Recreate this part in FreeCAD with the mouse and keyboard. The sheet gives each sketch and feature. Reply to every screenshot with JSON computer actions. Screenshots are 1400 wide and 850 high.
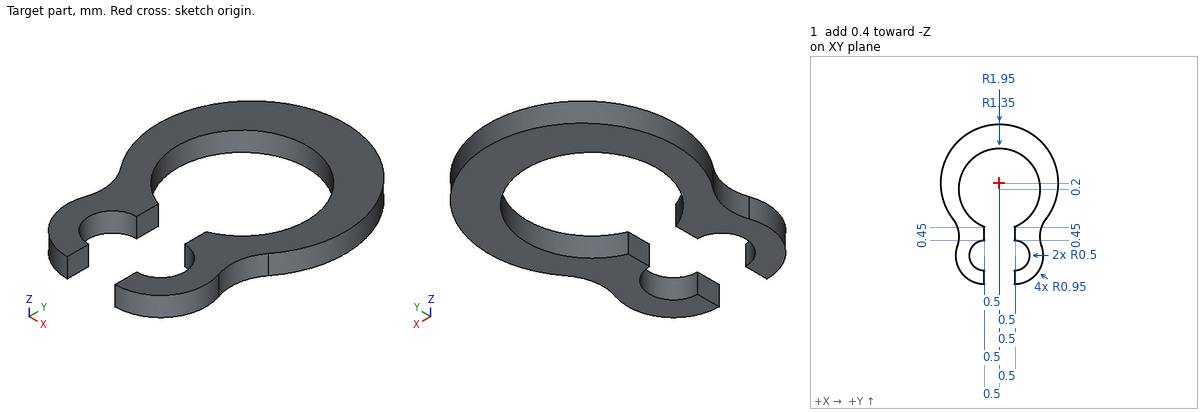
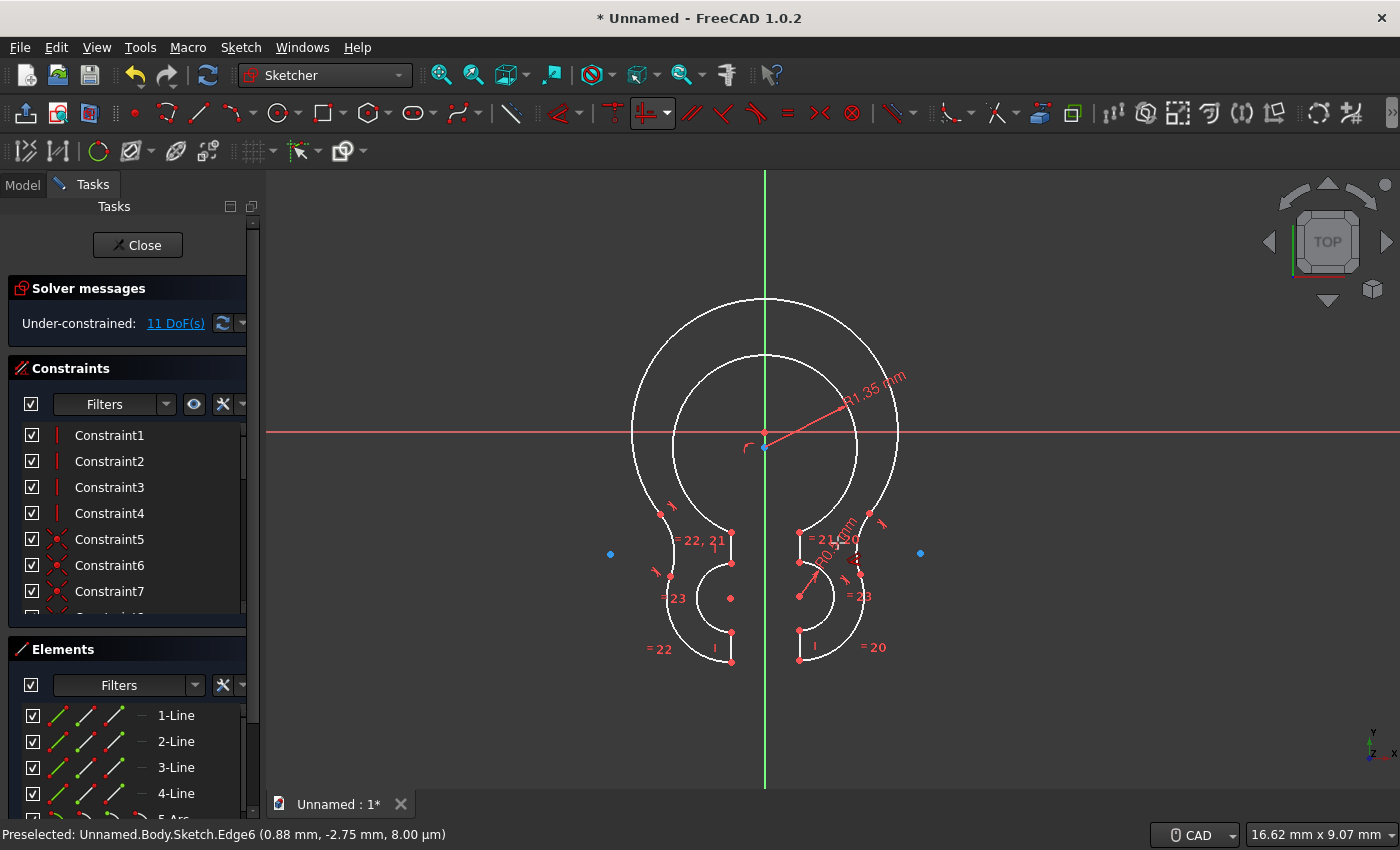
{"action": "left_click", "coordinate": [835, 650]}
{"action": "left_click", "coordinate": [853, 677]}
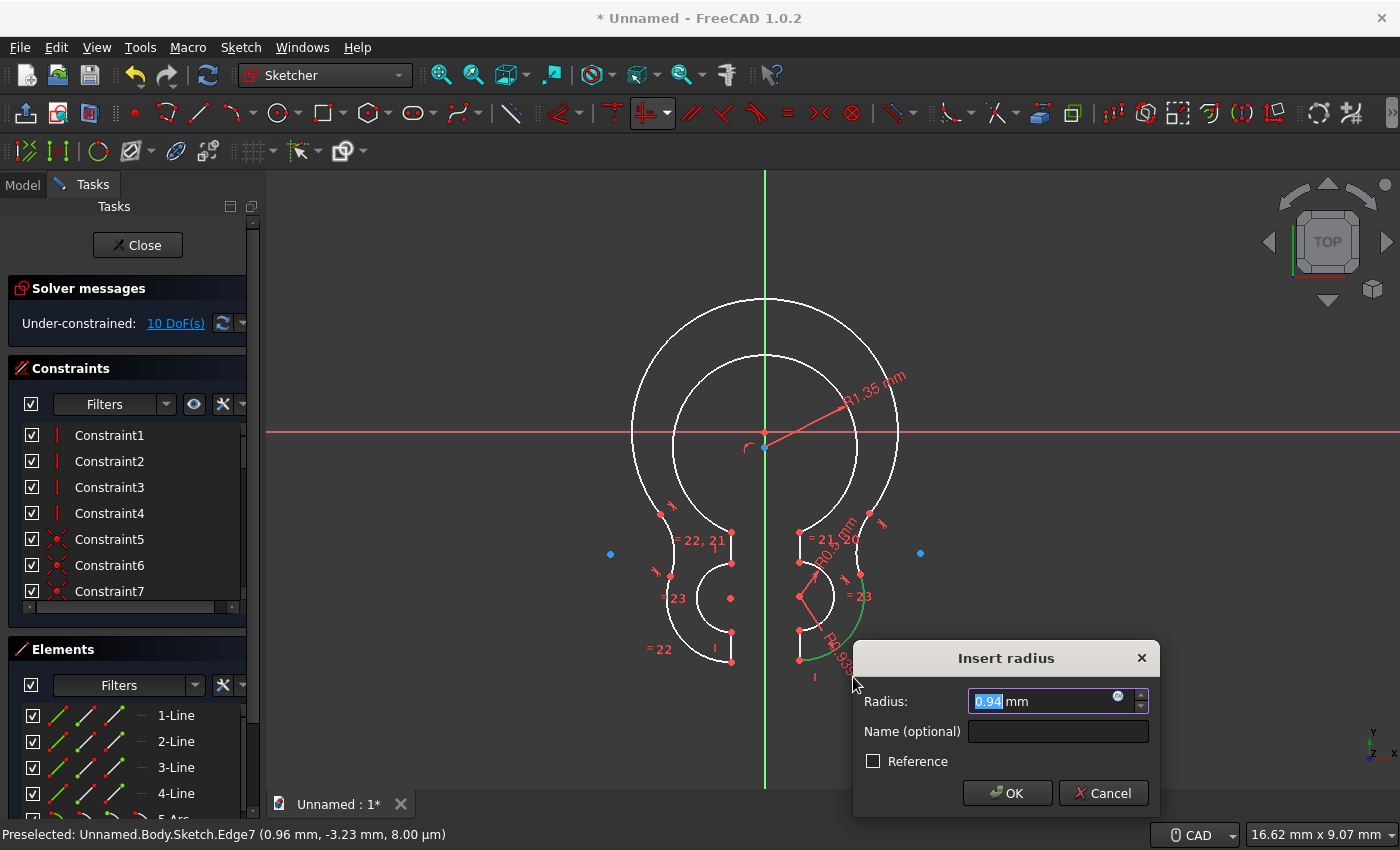
{"action": "type", "text": "0.95"}
{"action": "key", "text": "Return"}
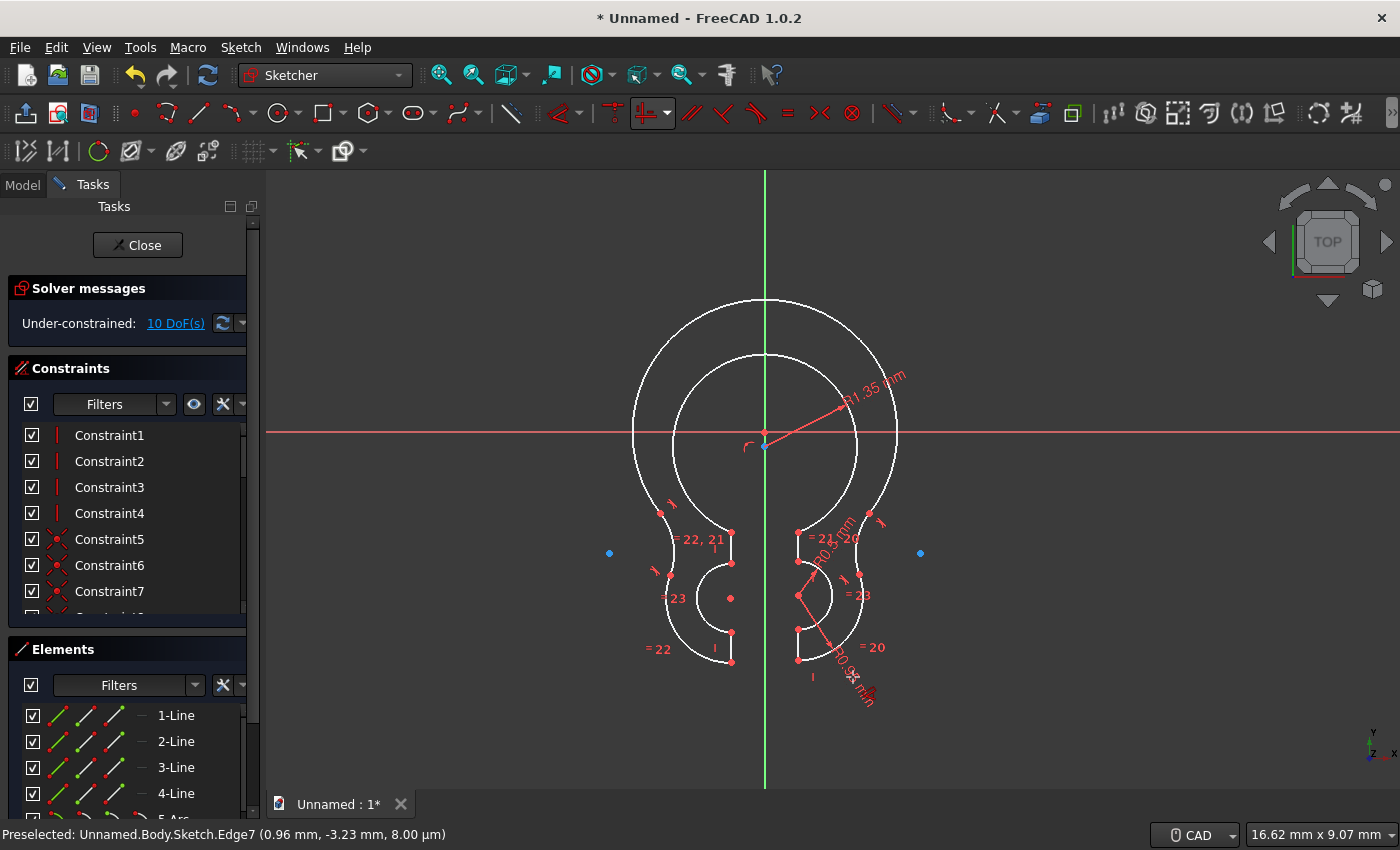
{"action": "left_click", "coordinate": [868, 349]}
{"action": "left_click", "coordinate": [893, 329]}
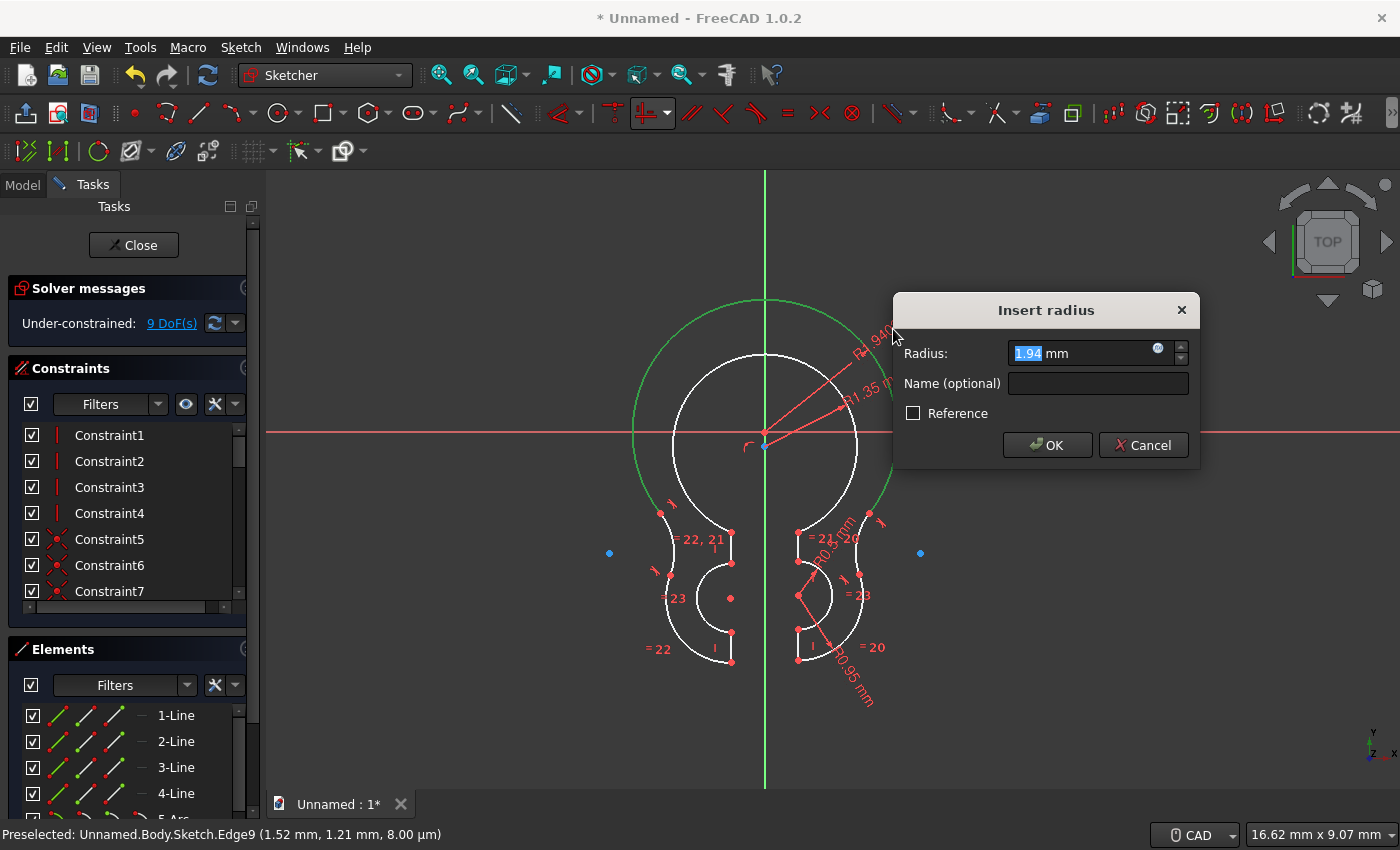
{"action": "type", "text": "1.95"}
{"action": "key", "text": "Return"}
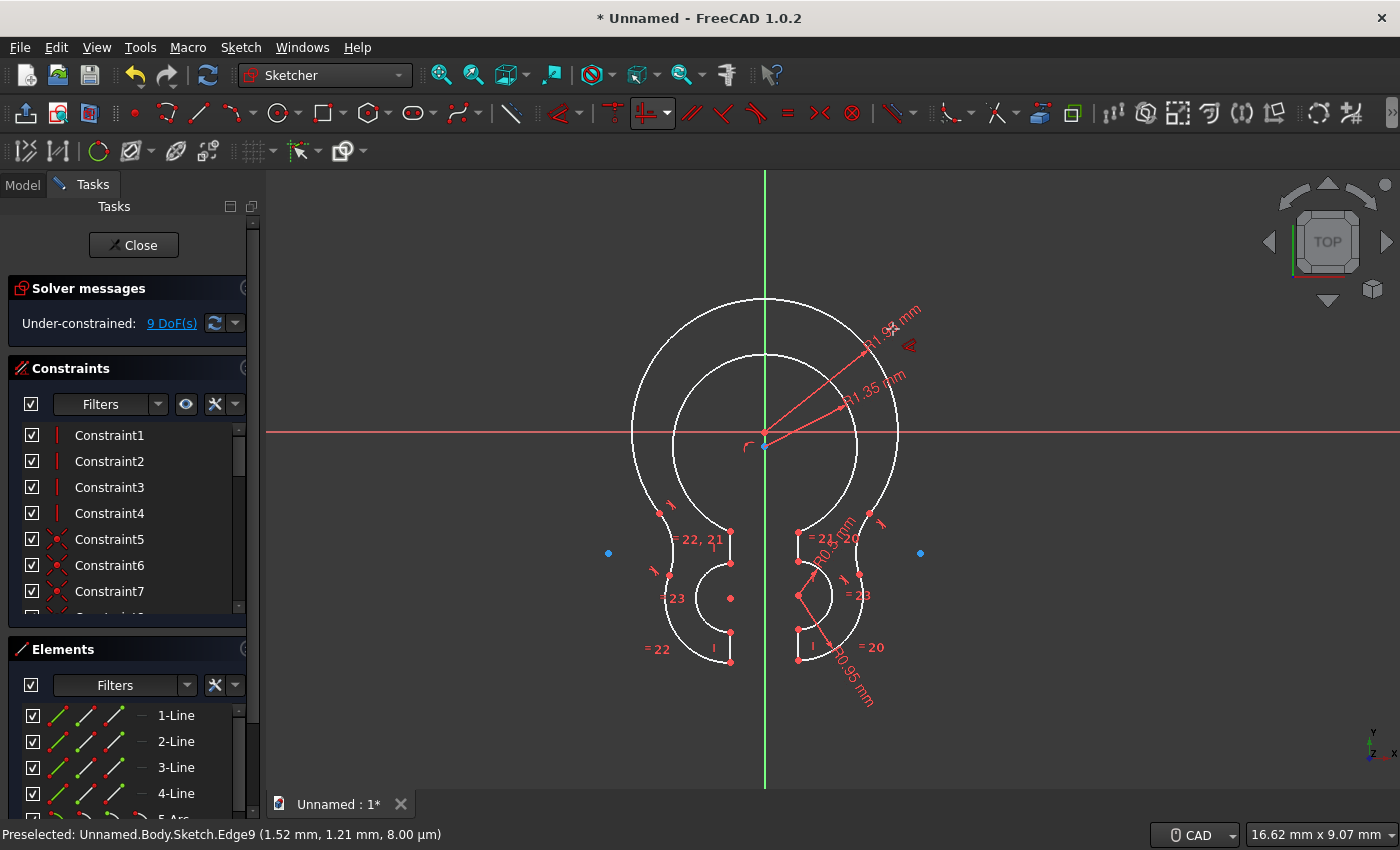
{"action": "scroll", "coordinate": [730, 554], "scroll_direction": "up", "scroll_amount": 2}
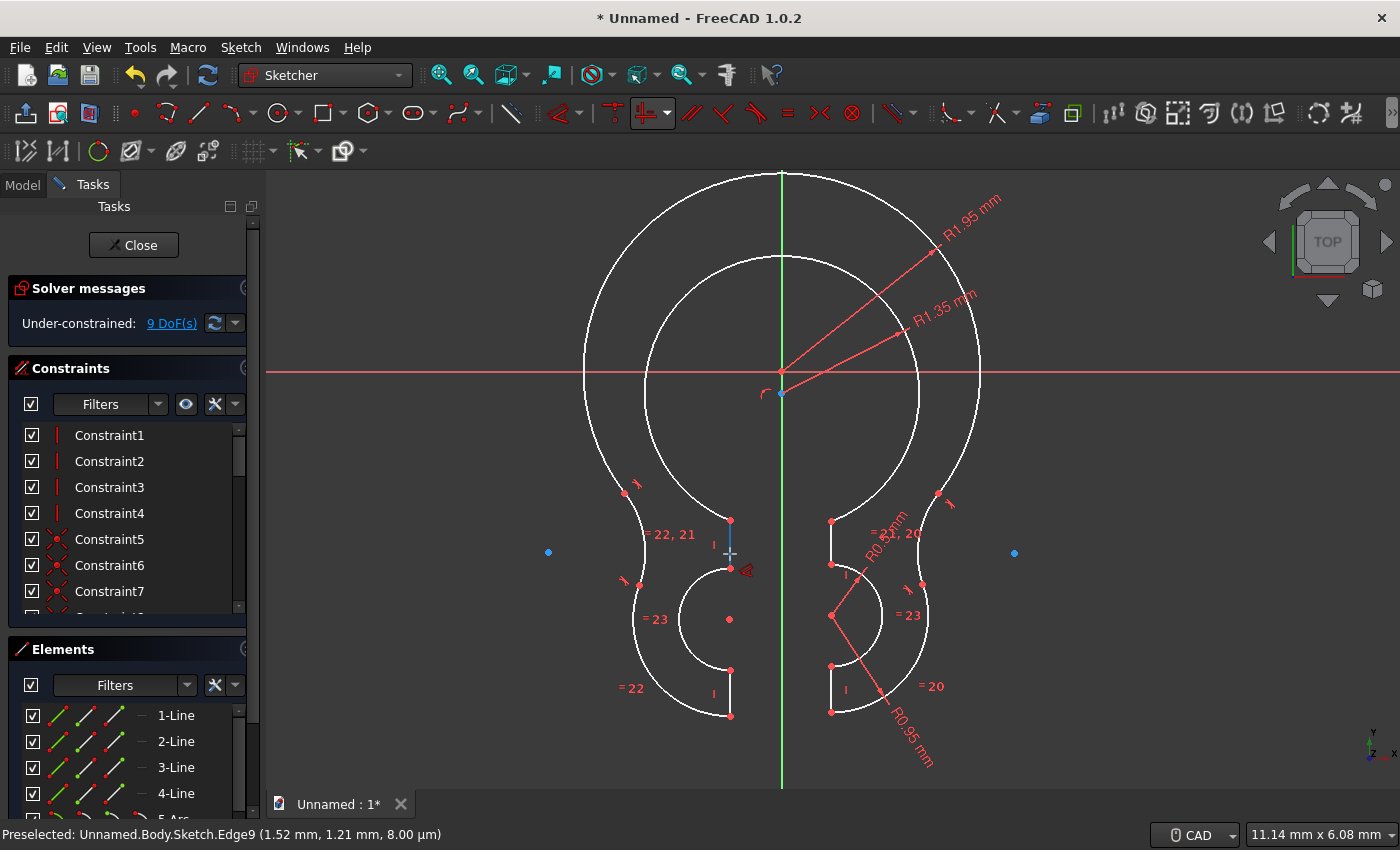
{"action": "left_click", "coordinate": [730, 554]}
{"action": "left_click", "coordinate": [696, 545]}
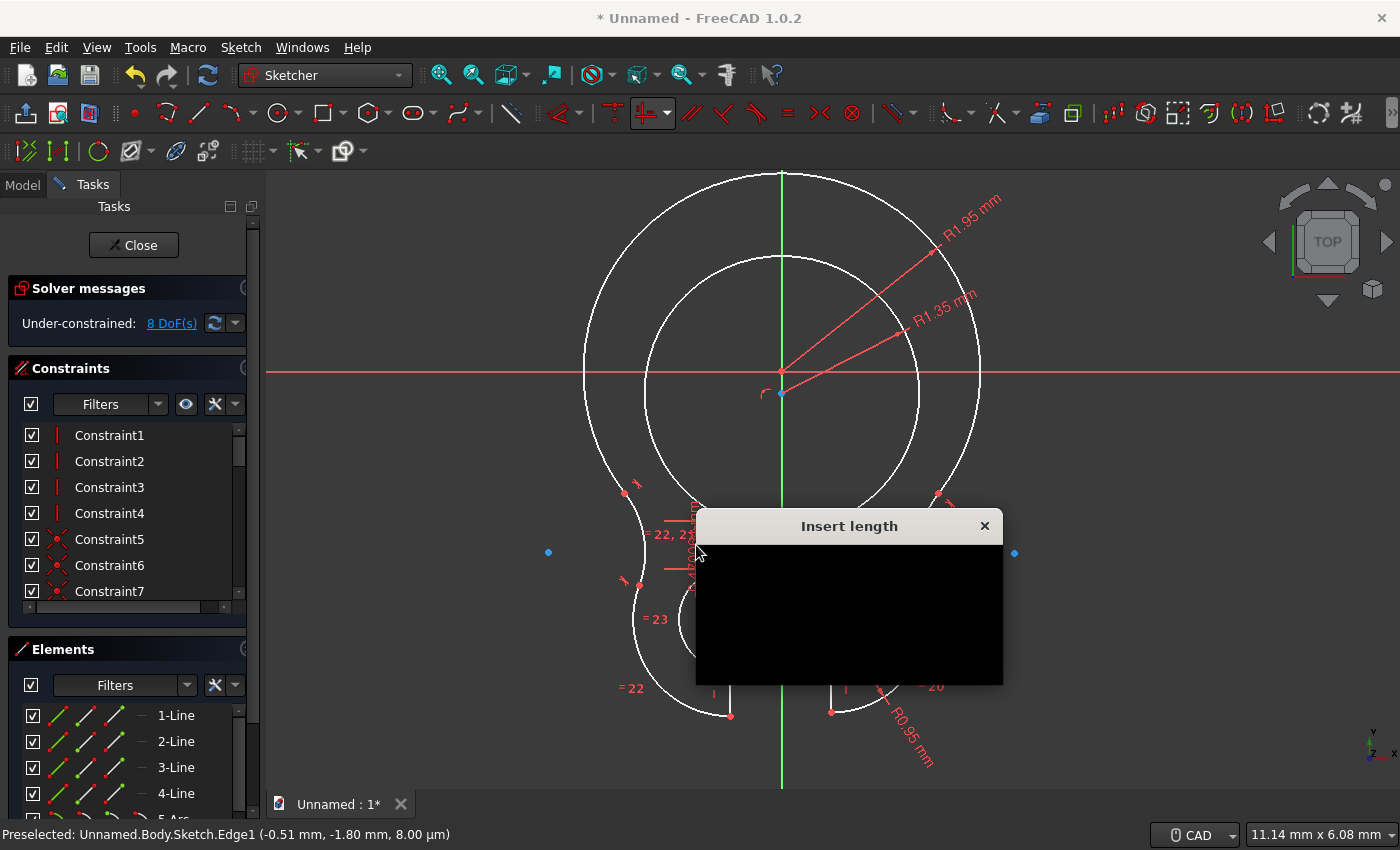
{"action": "type", "text": "0.45"}
{"action": "key", "text": "Return"}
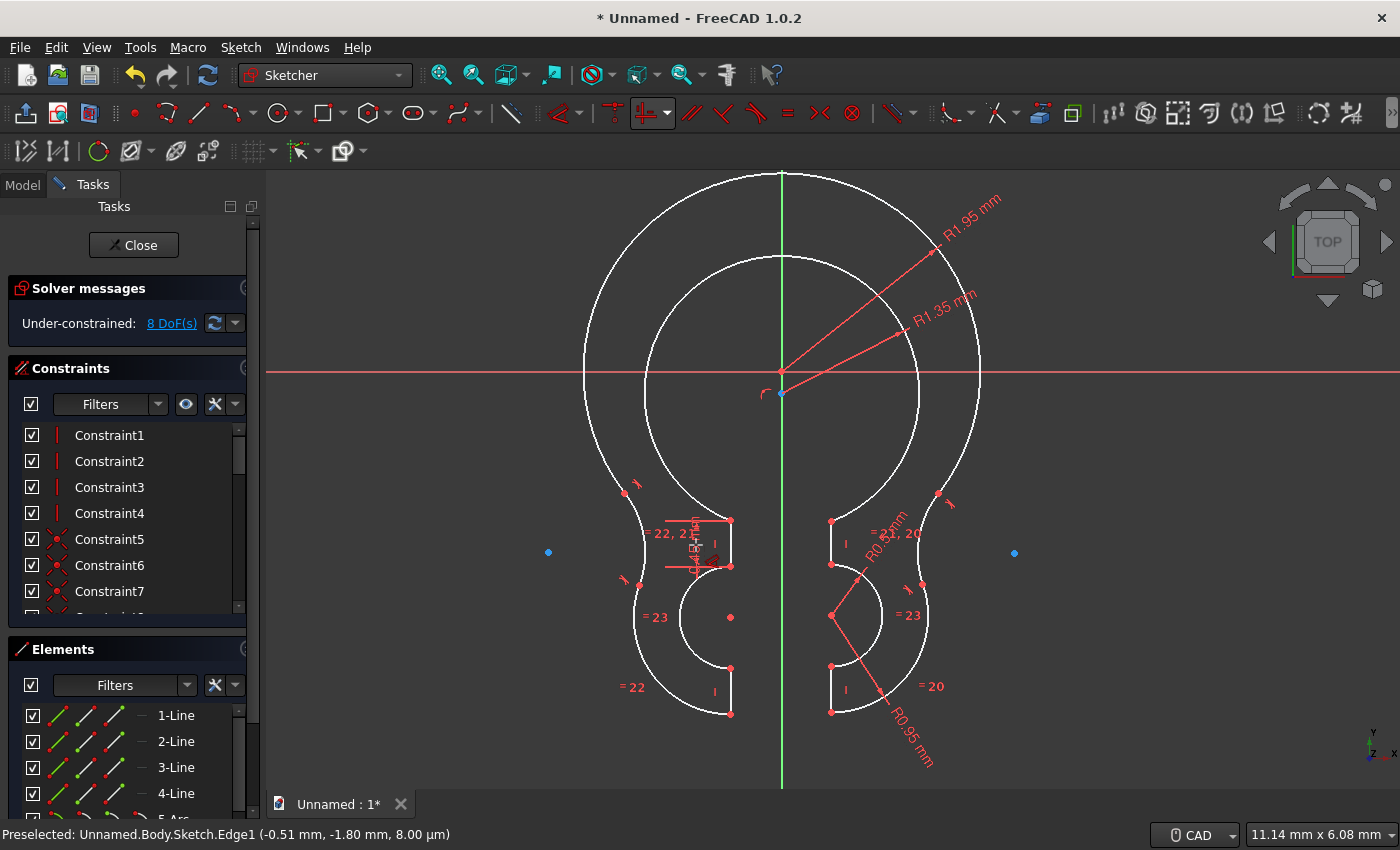
{"action": "left_click", "coordinate": [831, 535]}
{"action": "left_click", "coordinate": [865, 558]}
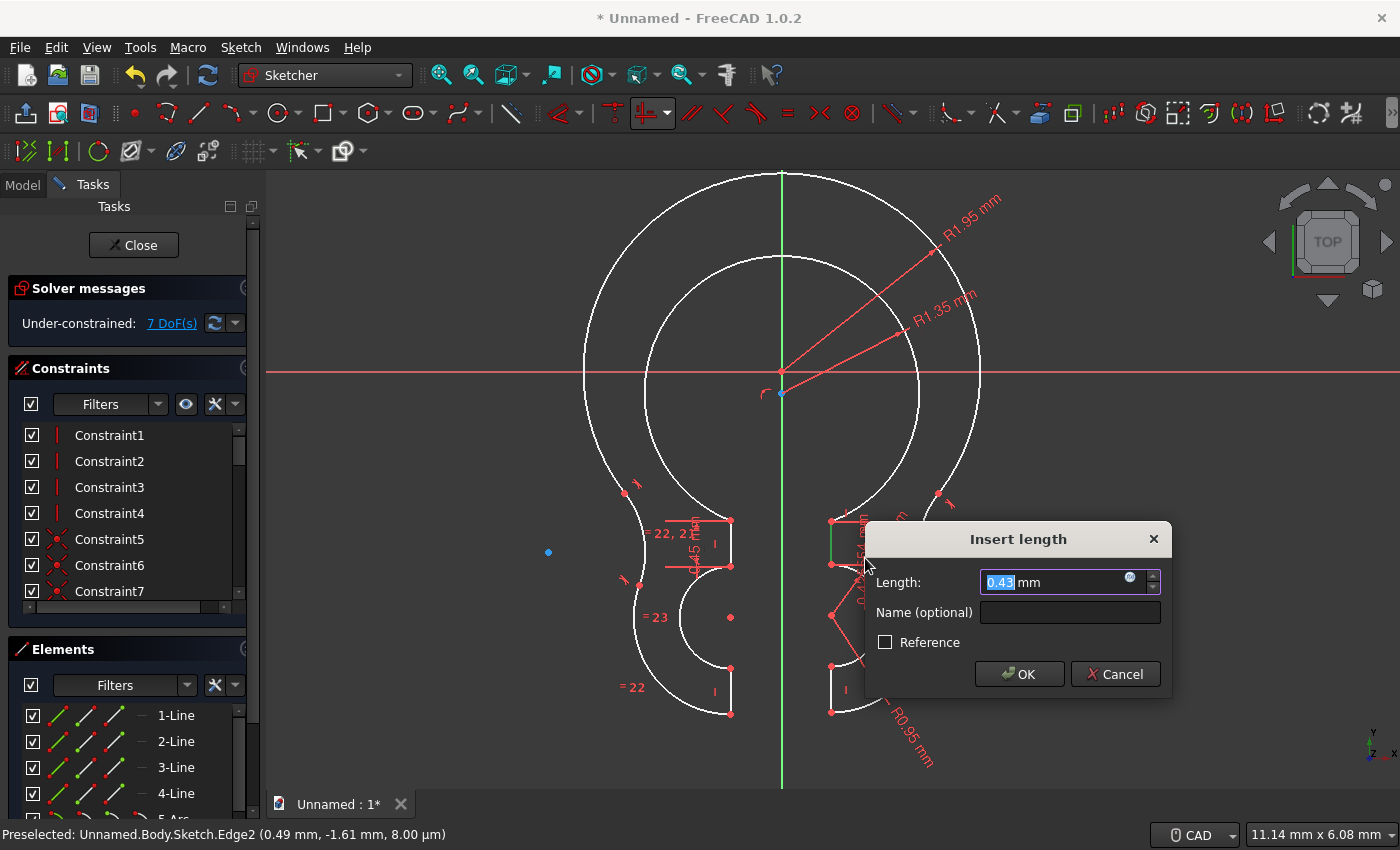
{"action": "type", "text": "0.45"}
{"action": "key", "text": "Return"}